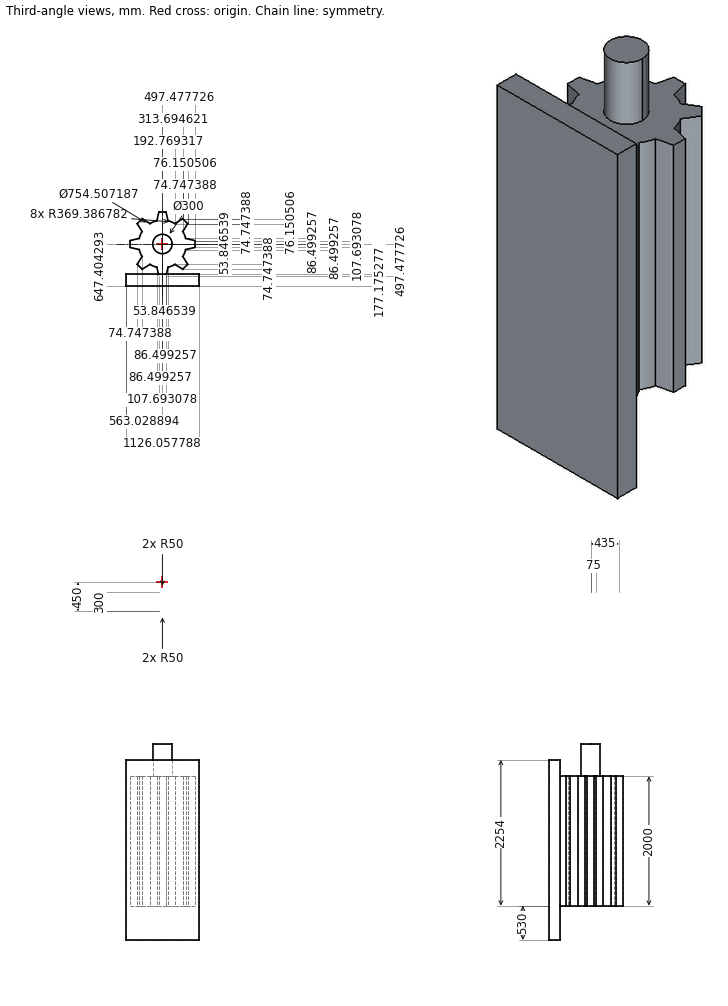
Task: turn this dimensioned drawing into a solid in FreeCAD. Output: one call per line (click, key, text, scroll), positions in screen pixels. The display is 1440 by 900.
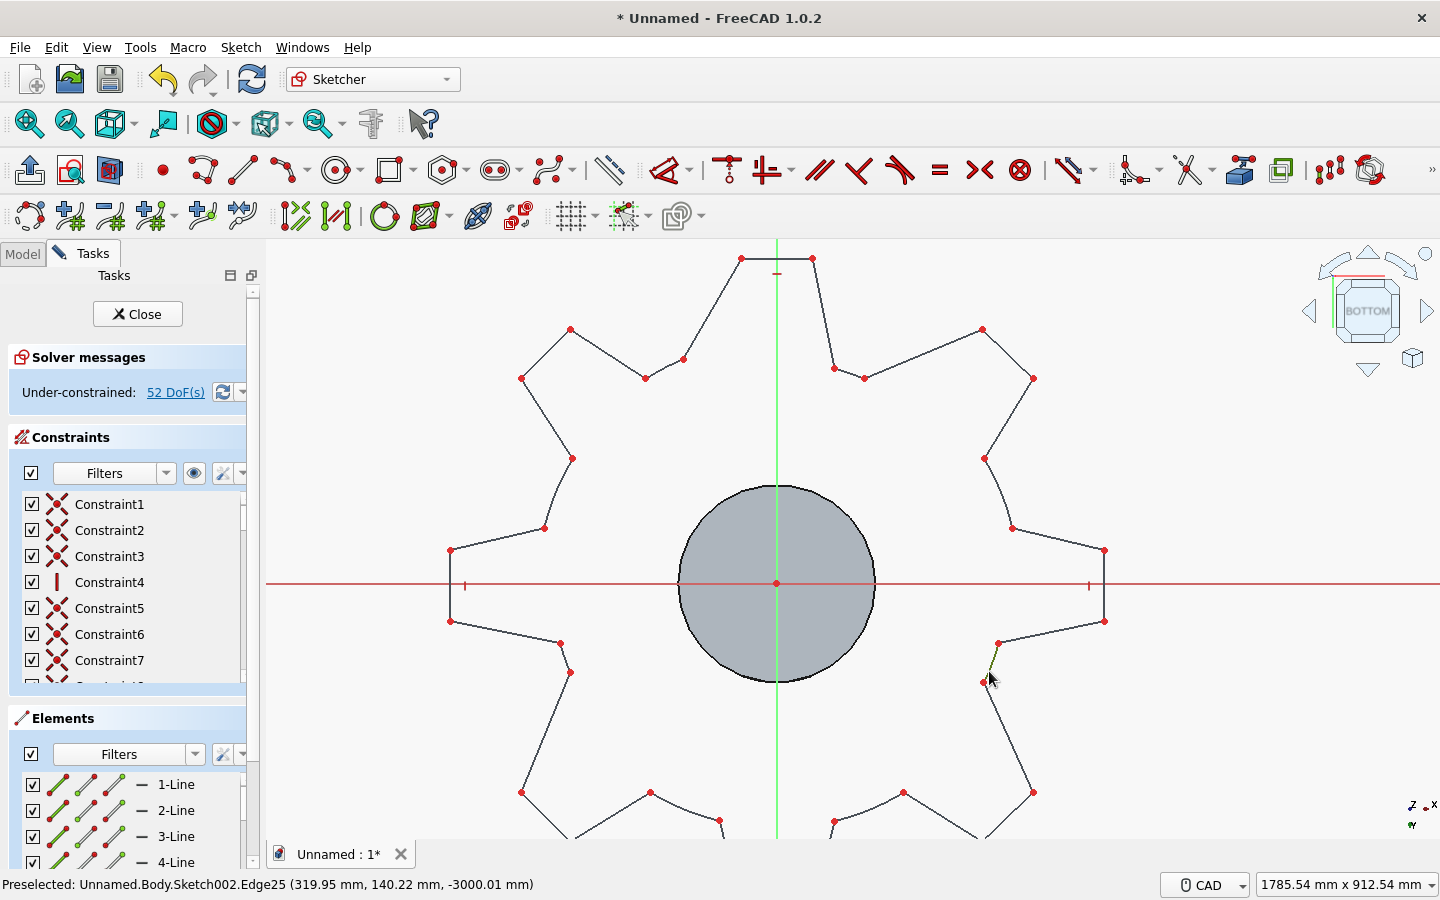
click(1006, 507)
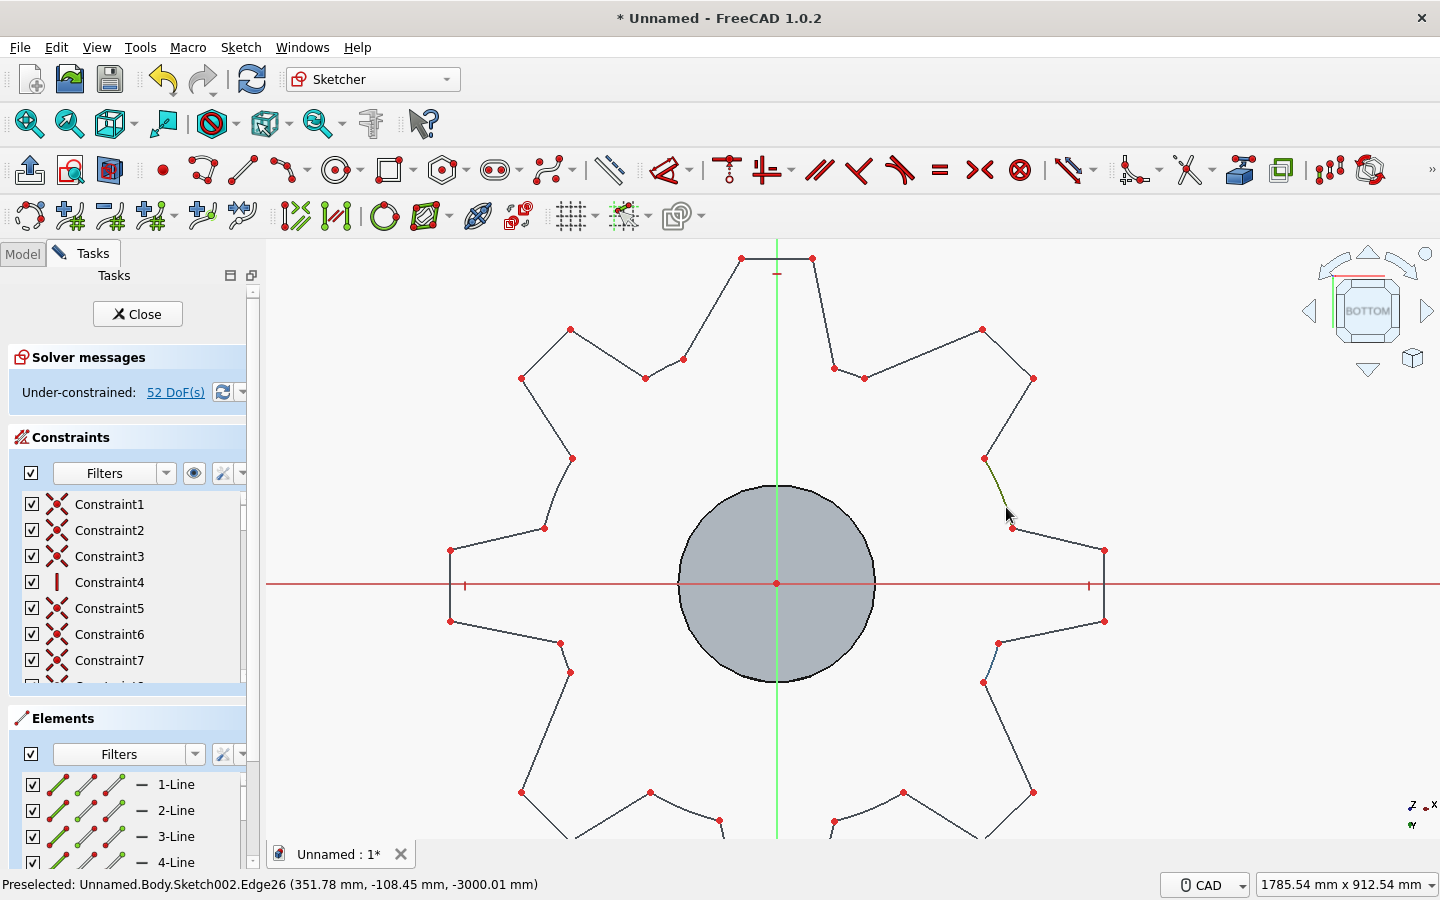
scroll(855, 375, up, 2)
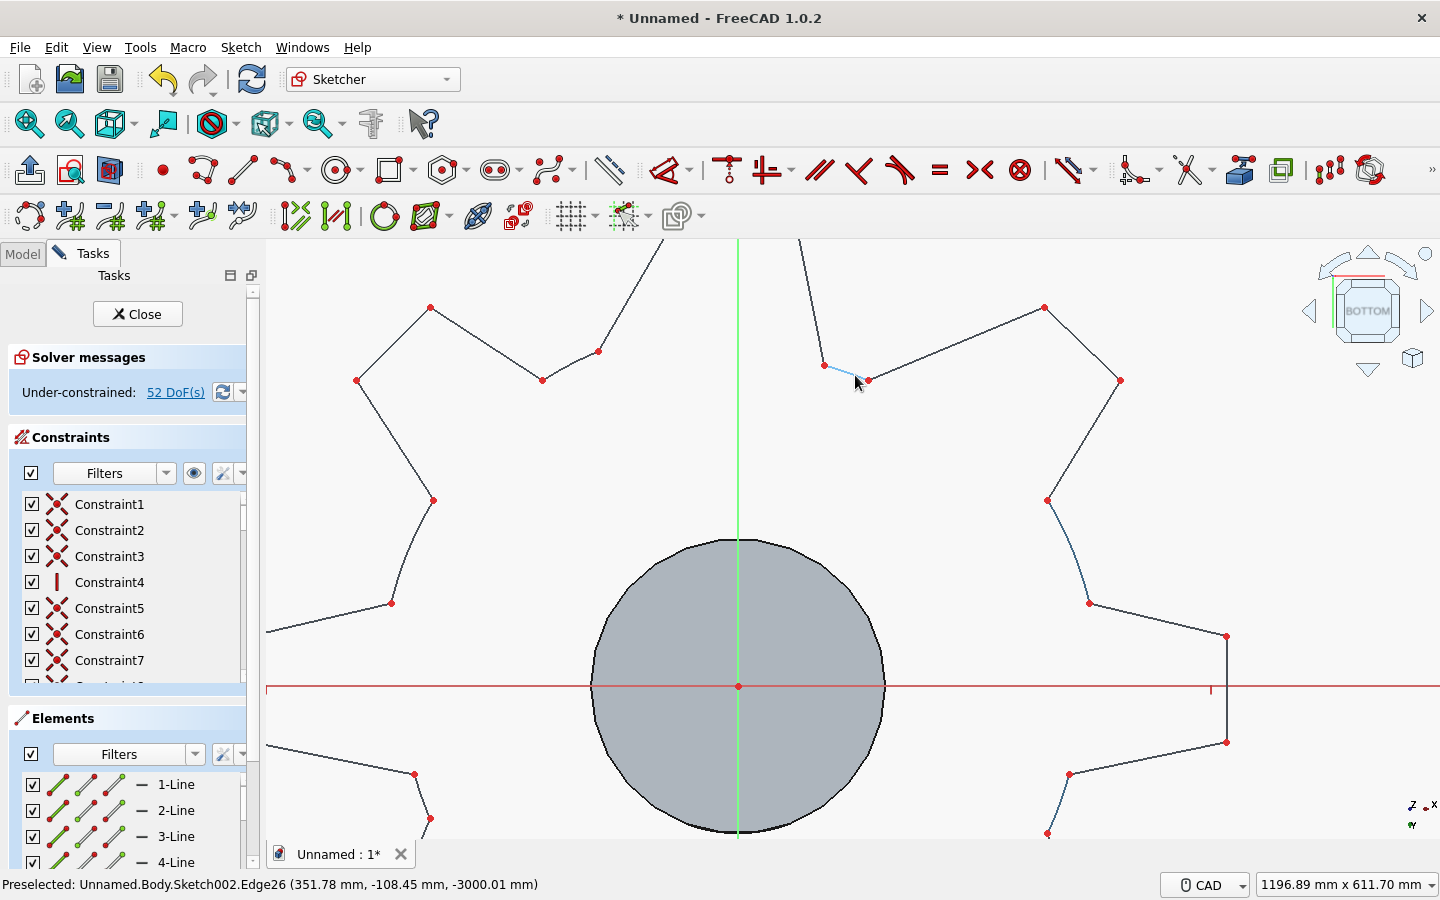
click(855, 375)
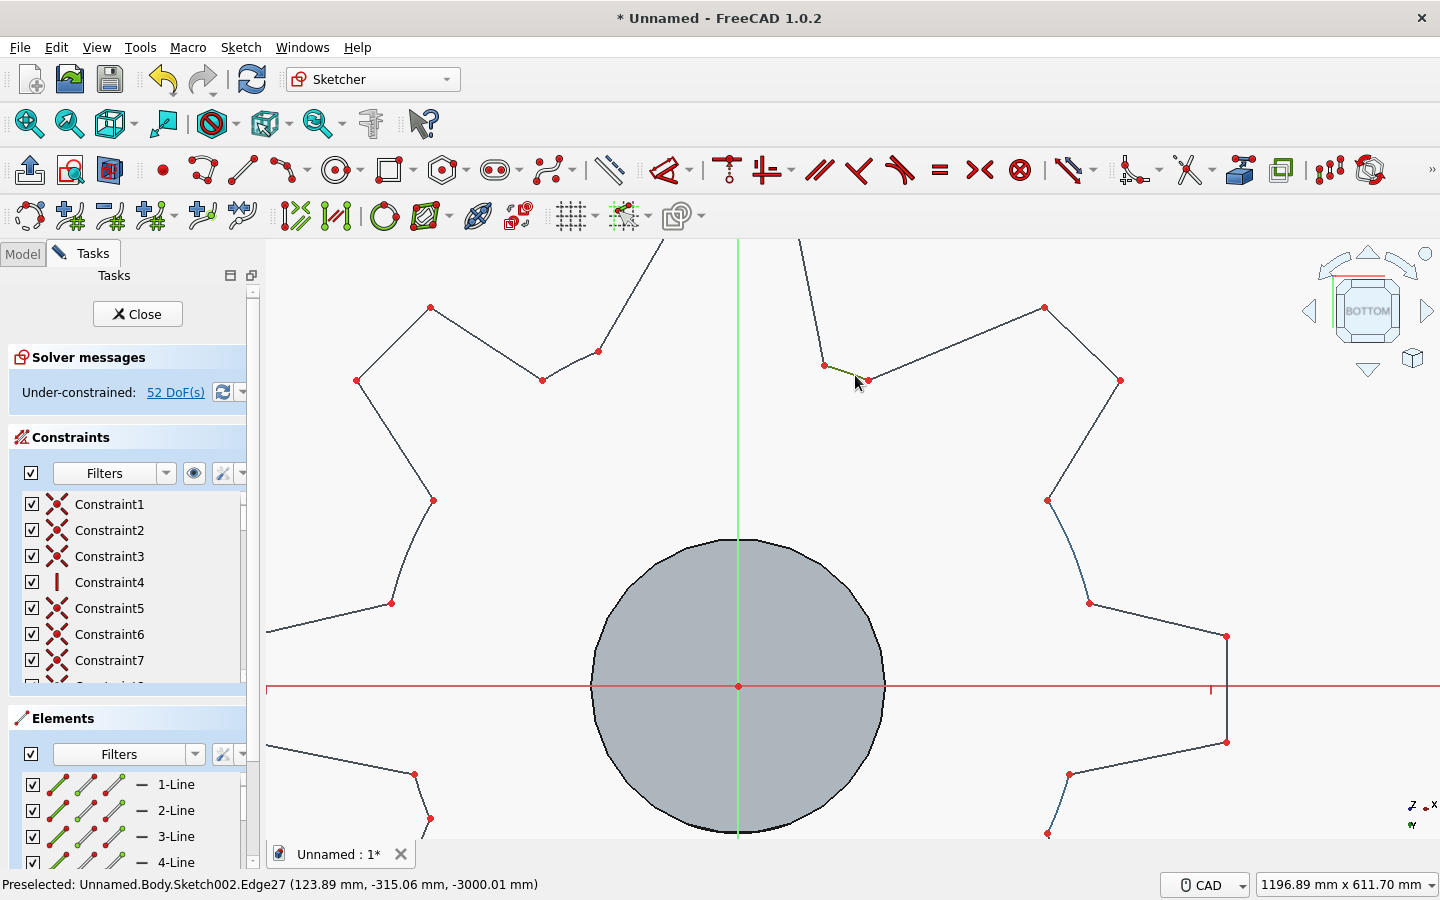
click(581, 359)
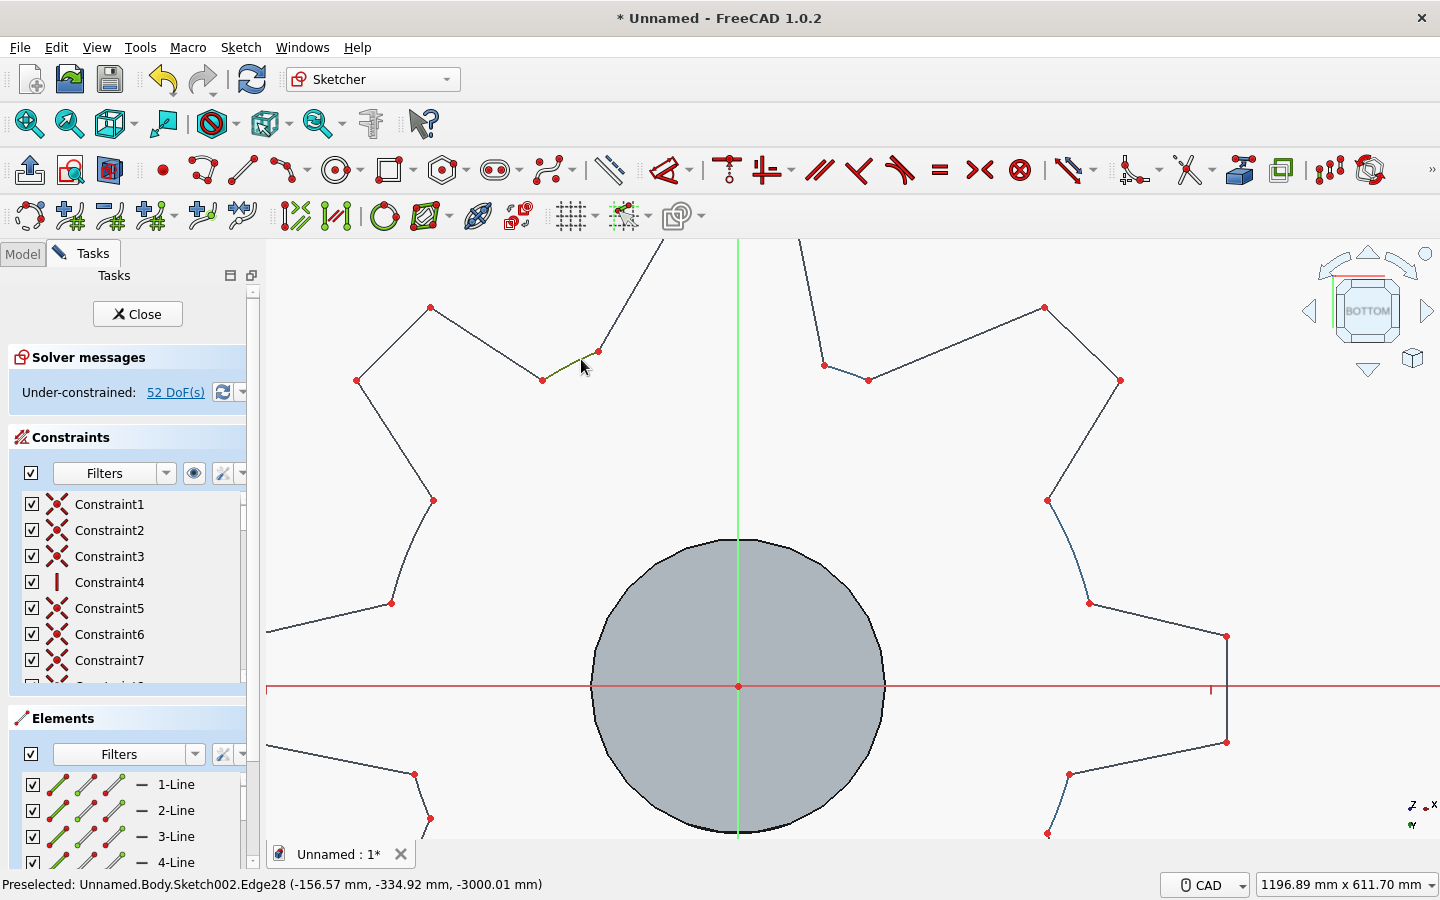
click(418, 530)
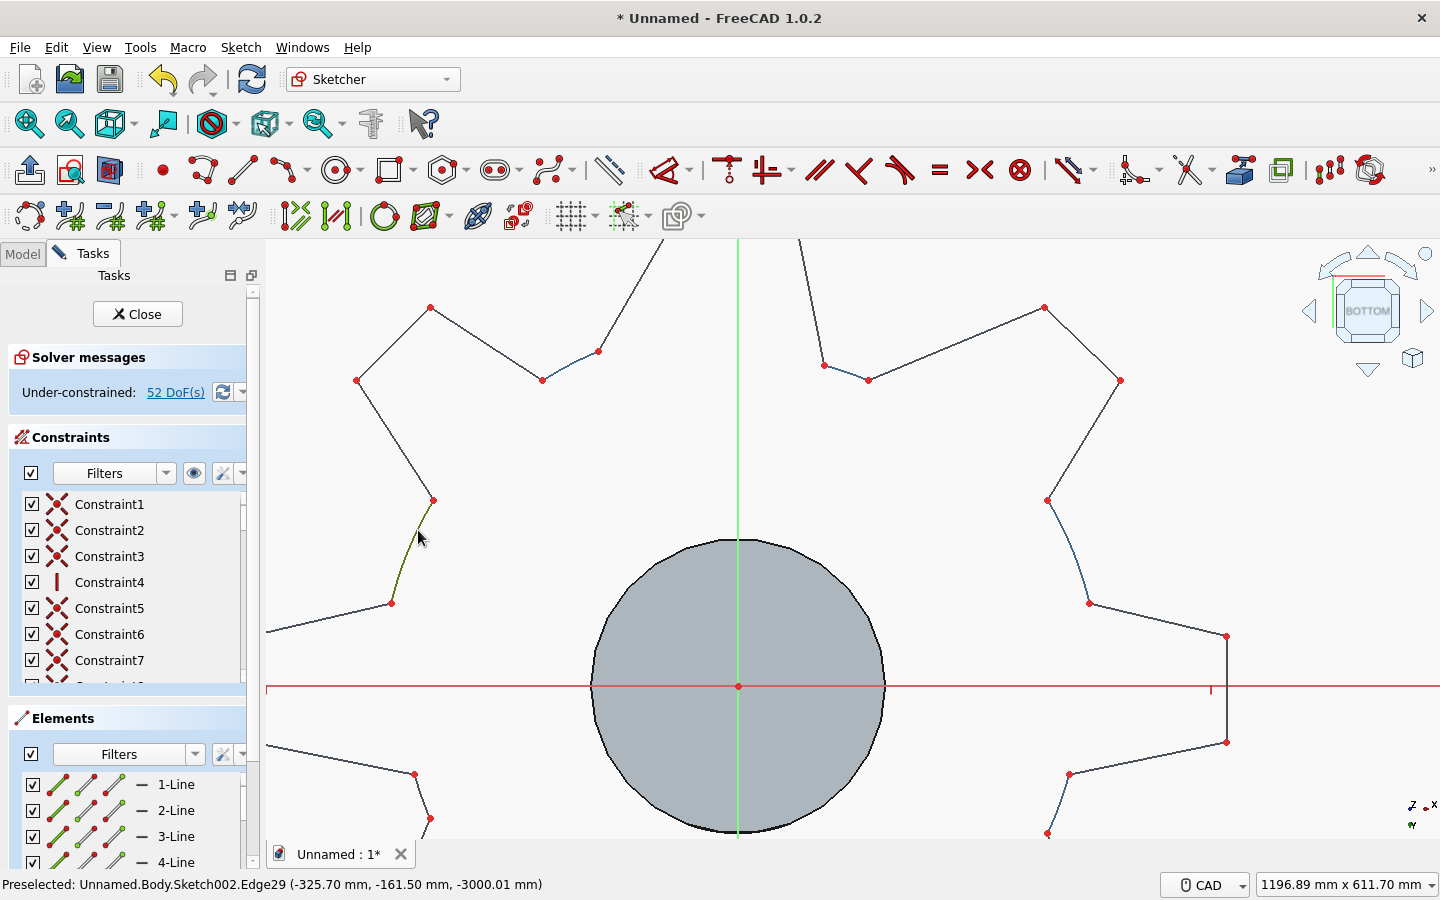
click(419, 788)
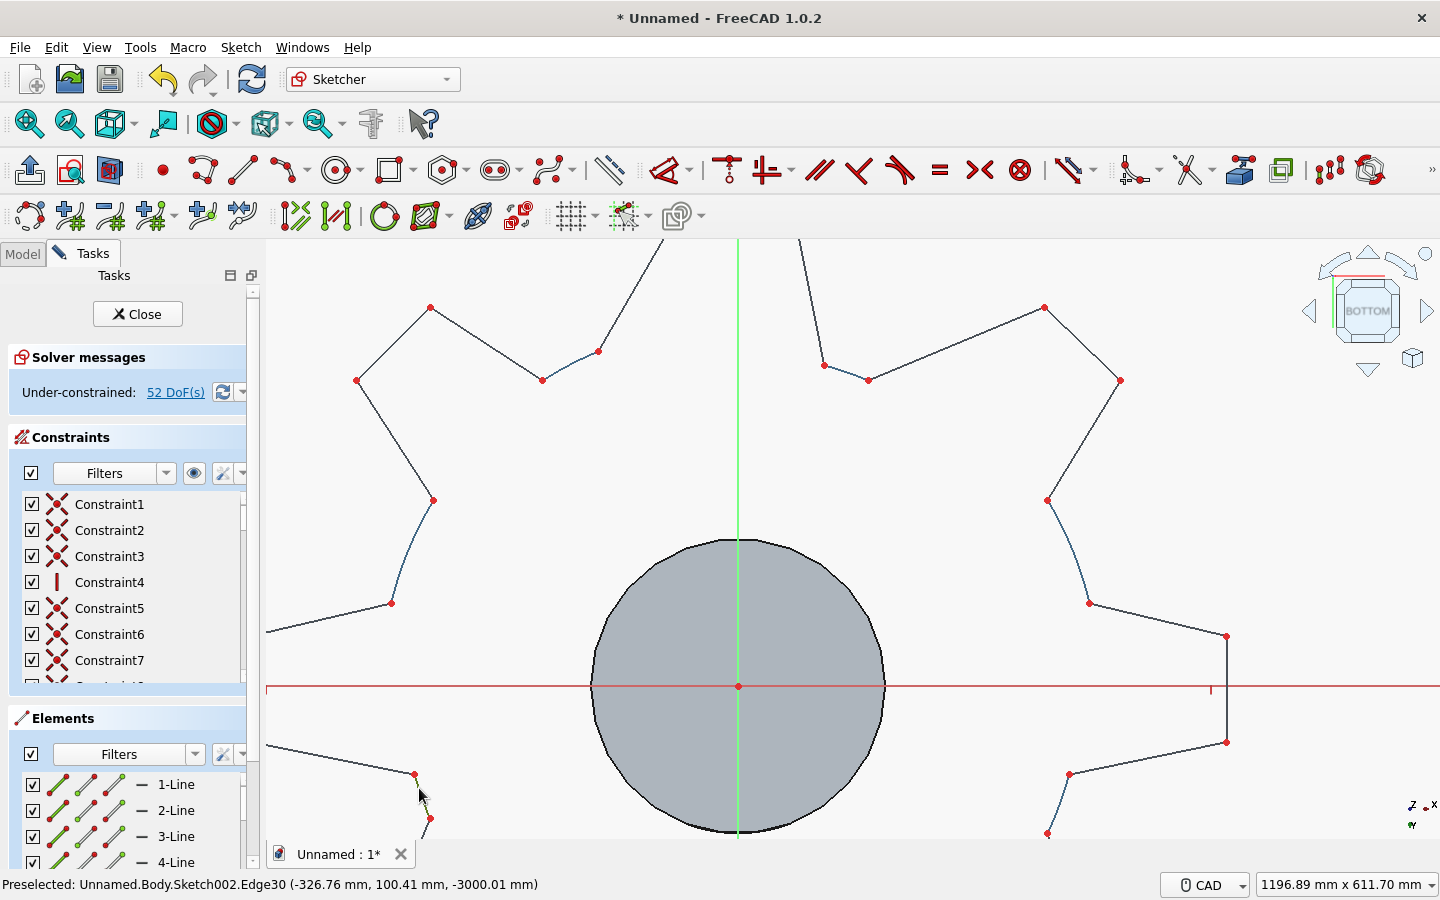
scroll(812, 453, down, 5)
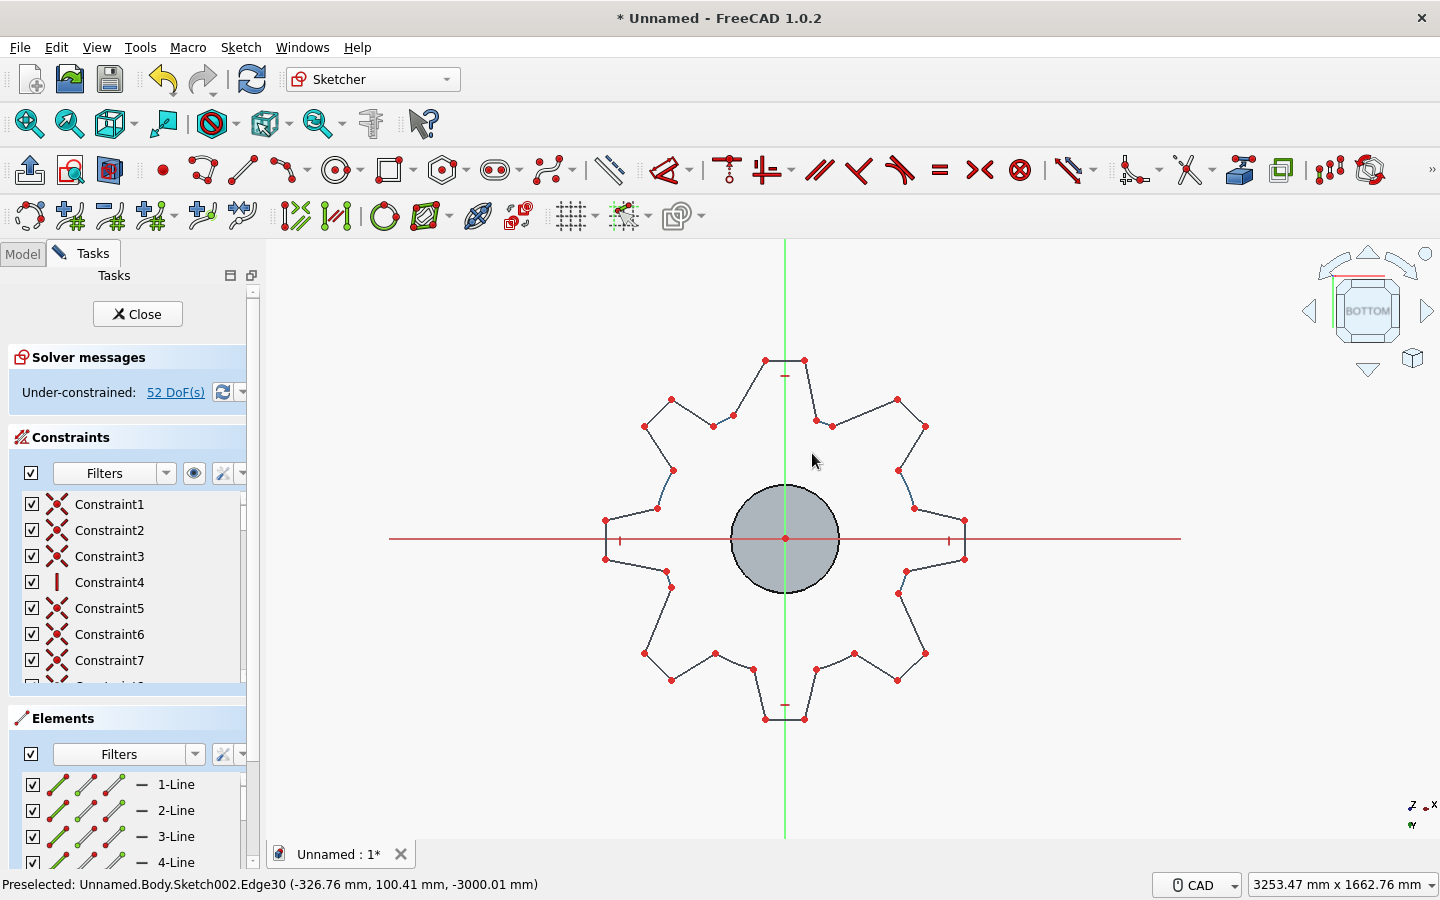
click(727, 659)